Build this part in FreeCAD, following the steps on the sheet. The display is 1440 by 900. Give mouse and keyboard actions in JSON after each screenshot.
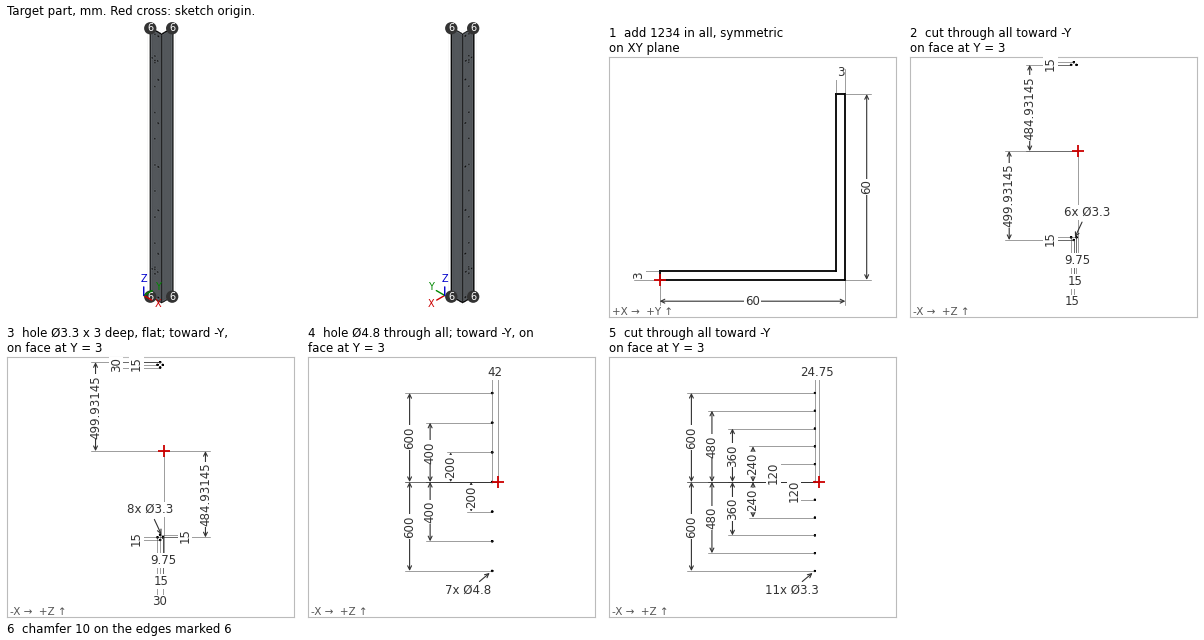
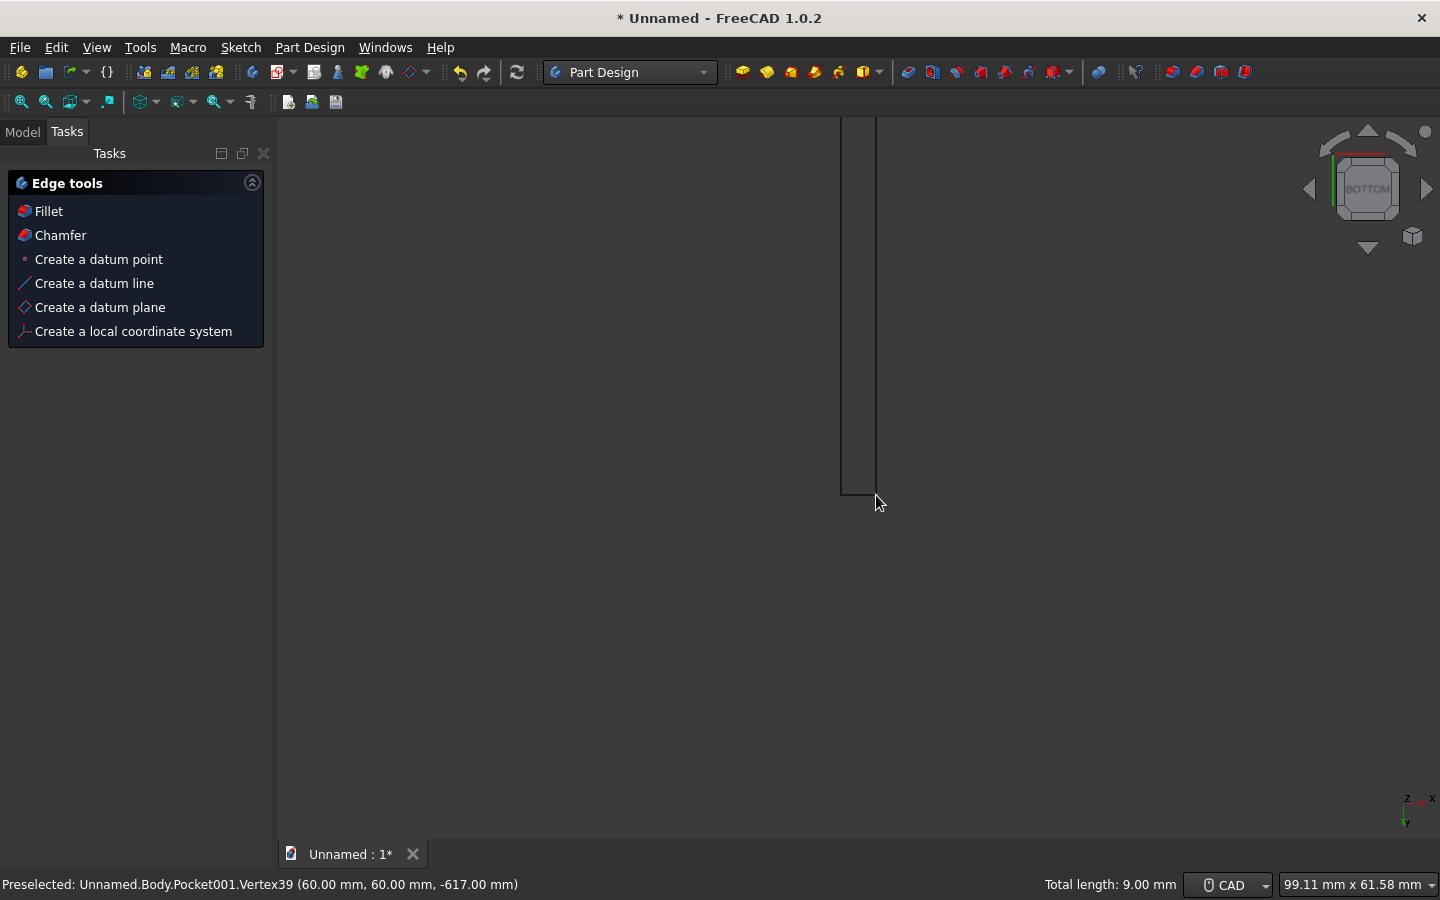
{"action": "left_click", "coordinate": [859, 494], "text": "ctrl"}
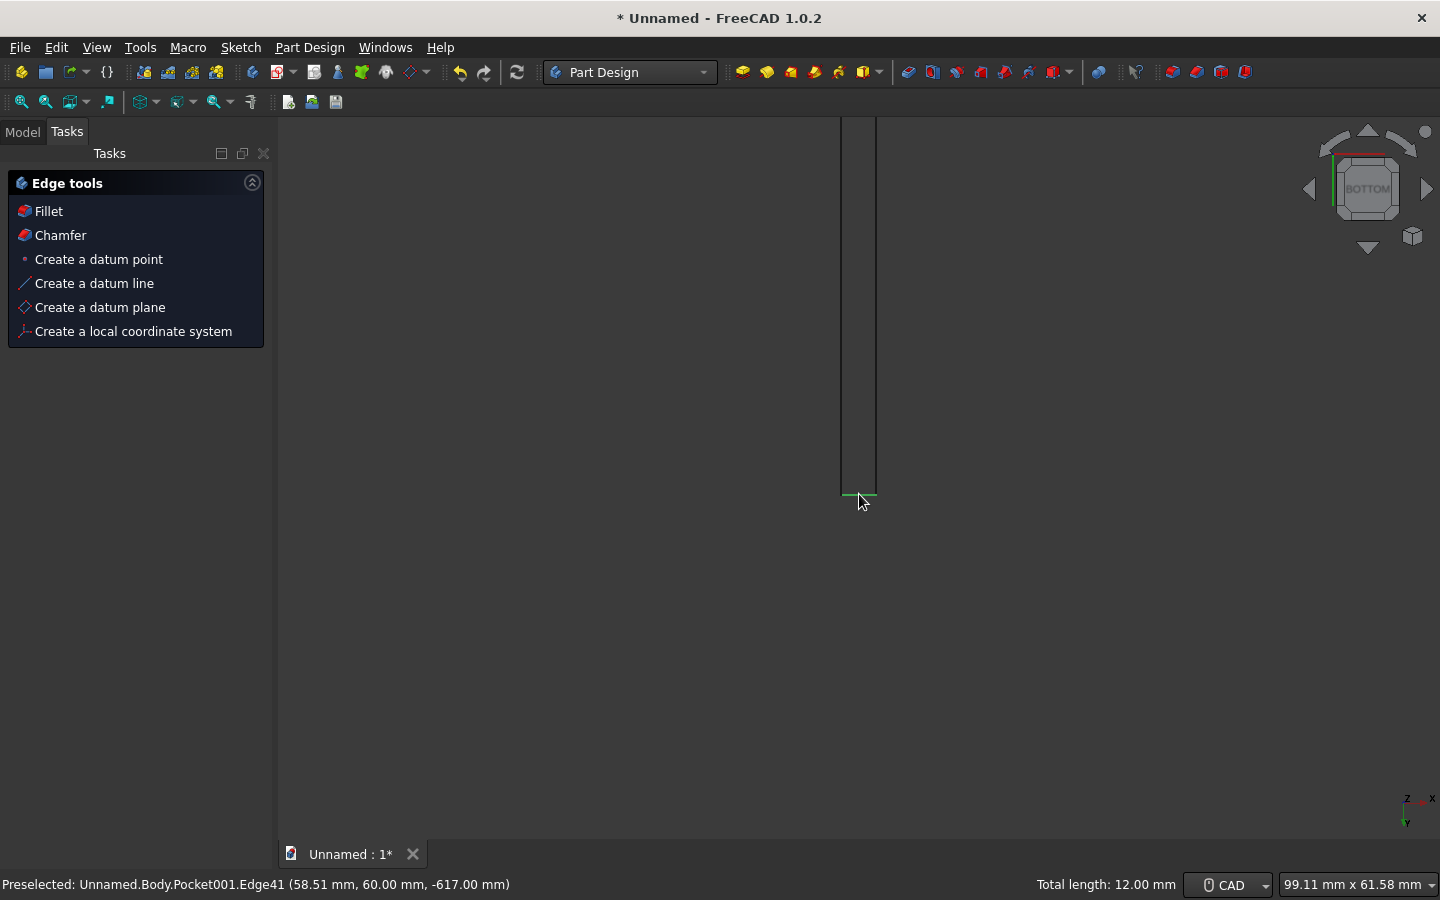
{"action": "key", "text": "v 1"}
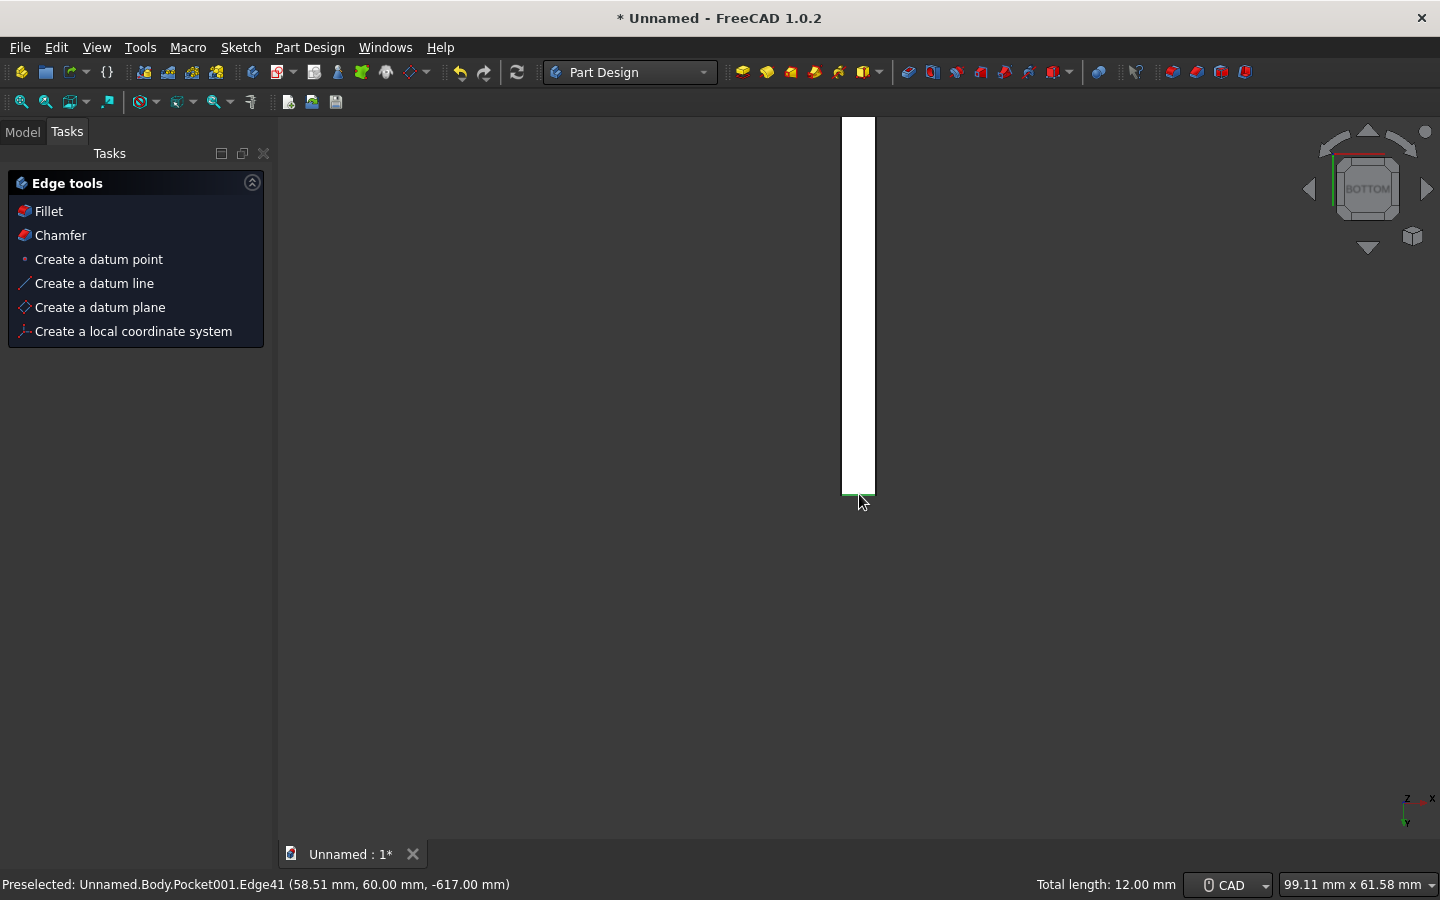
{"action": "left_click", "coordinate": [1198, 72]}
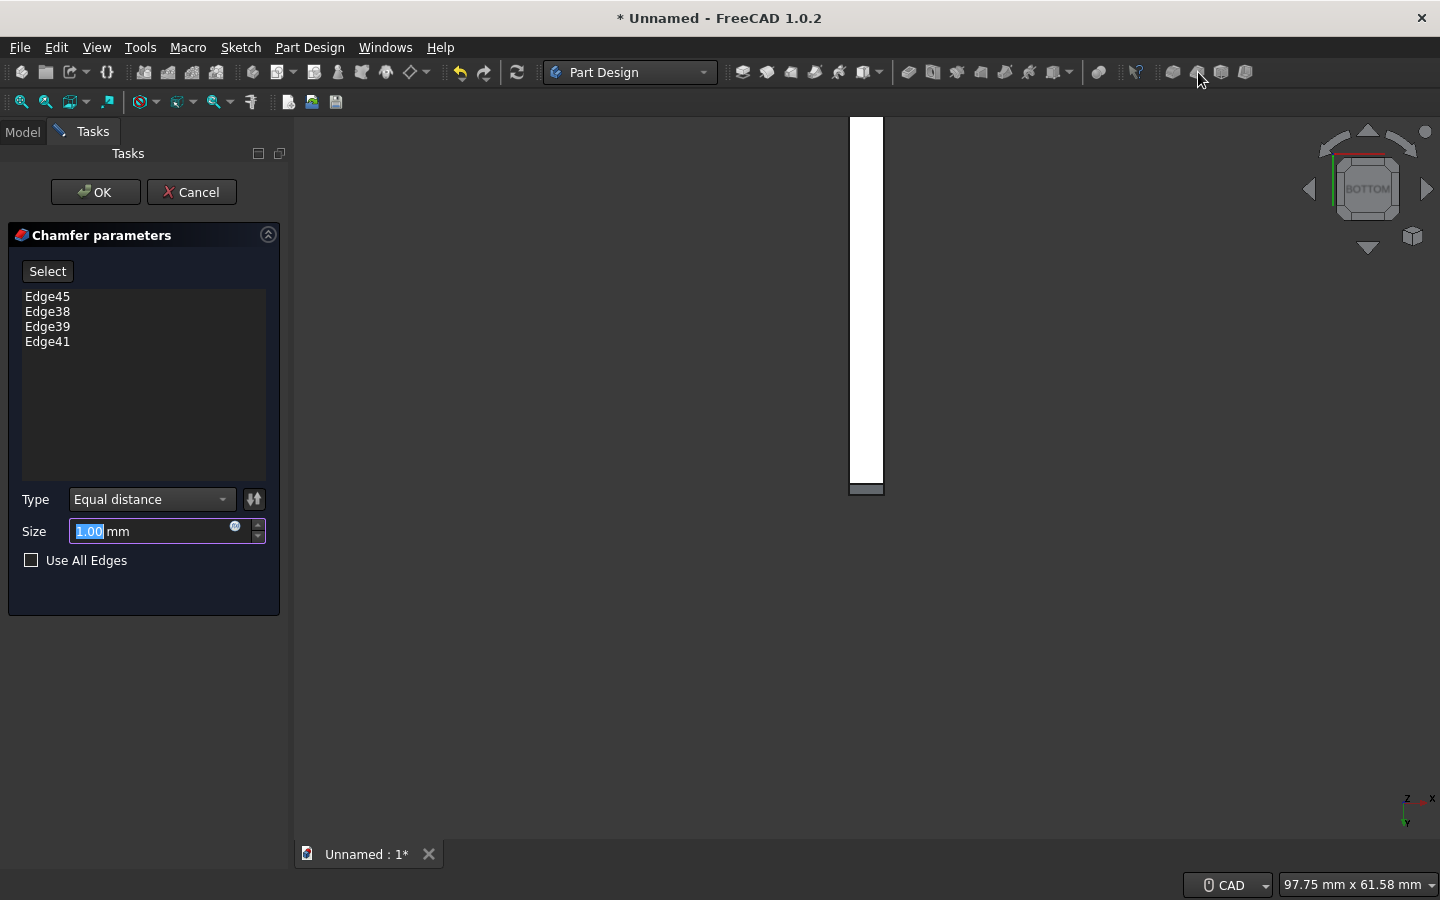
{"action": "type", "text": "10"}
{"action": "key", "text": "Tab"}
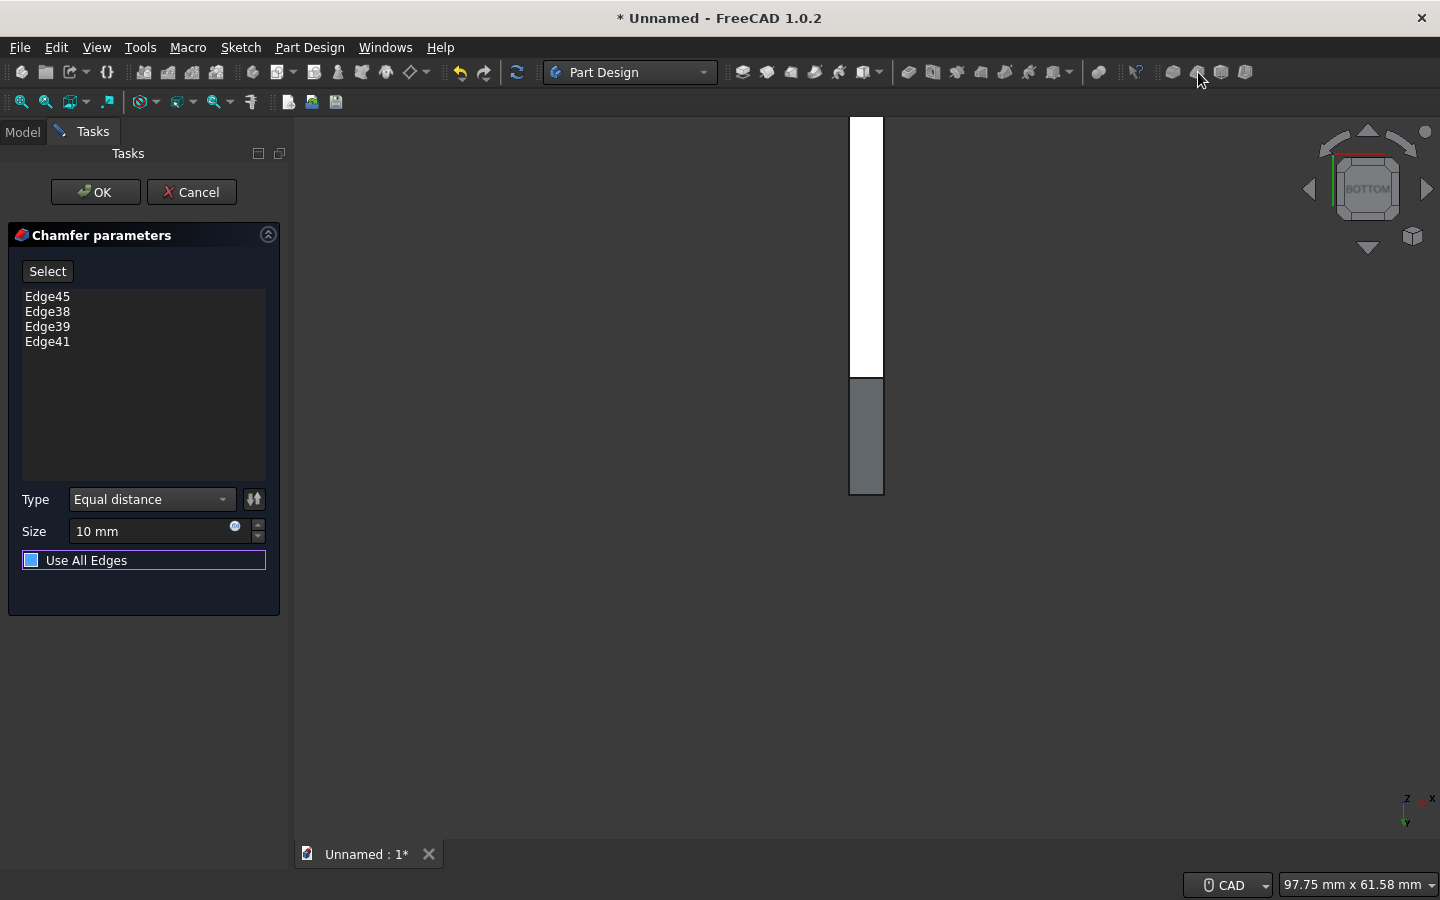
{"action": "left_click", "coordinate": [96, 192]}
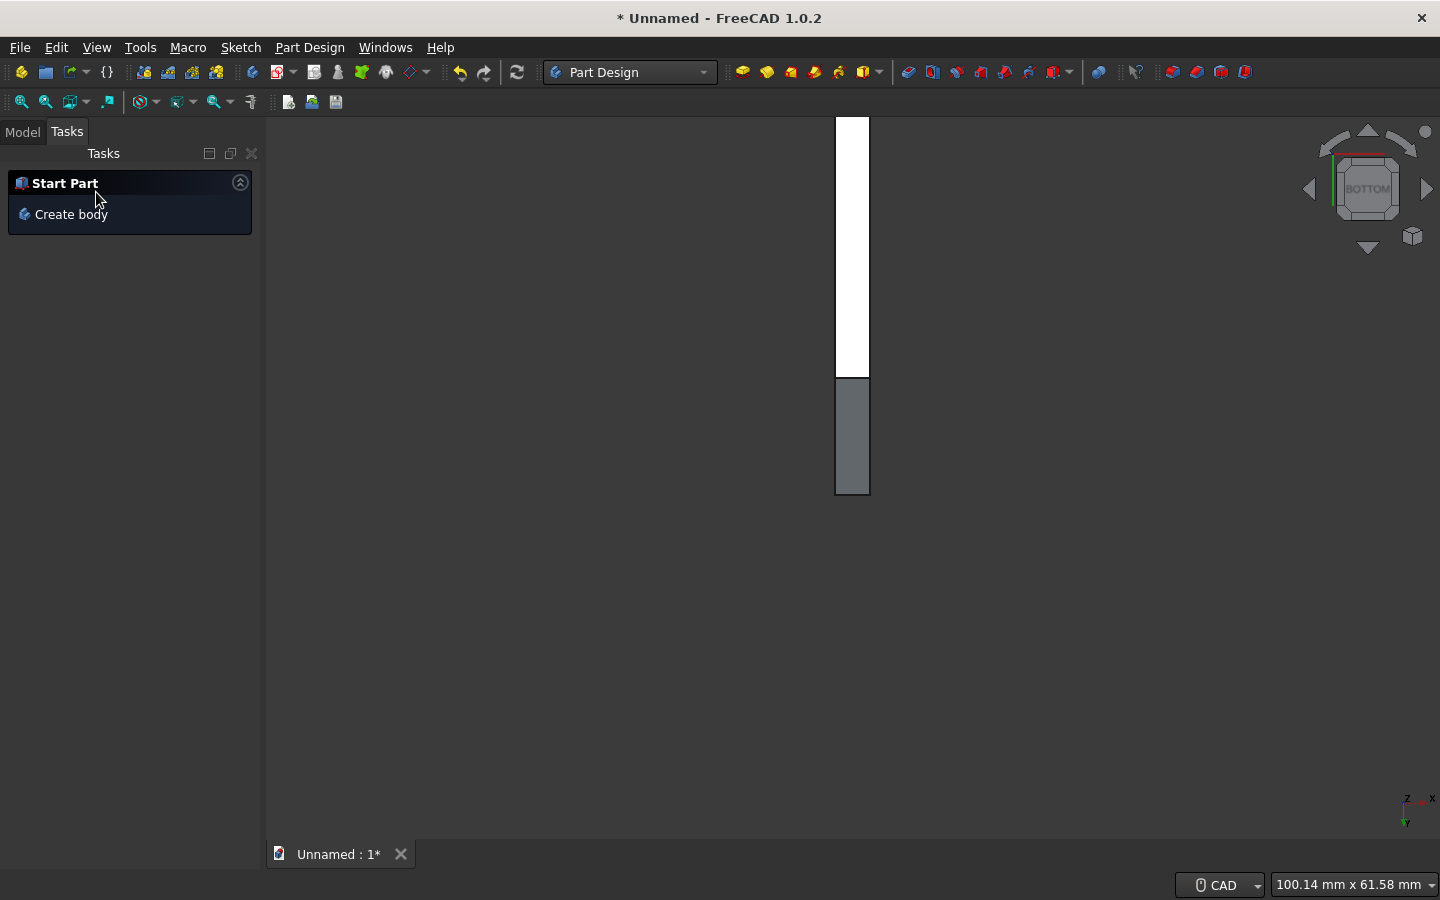
{"action": "key", "text": "0"}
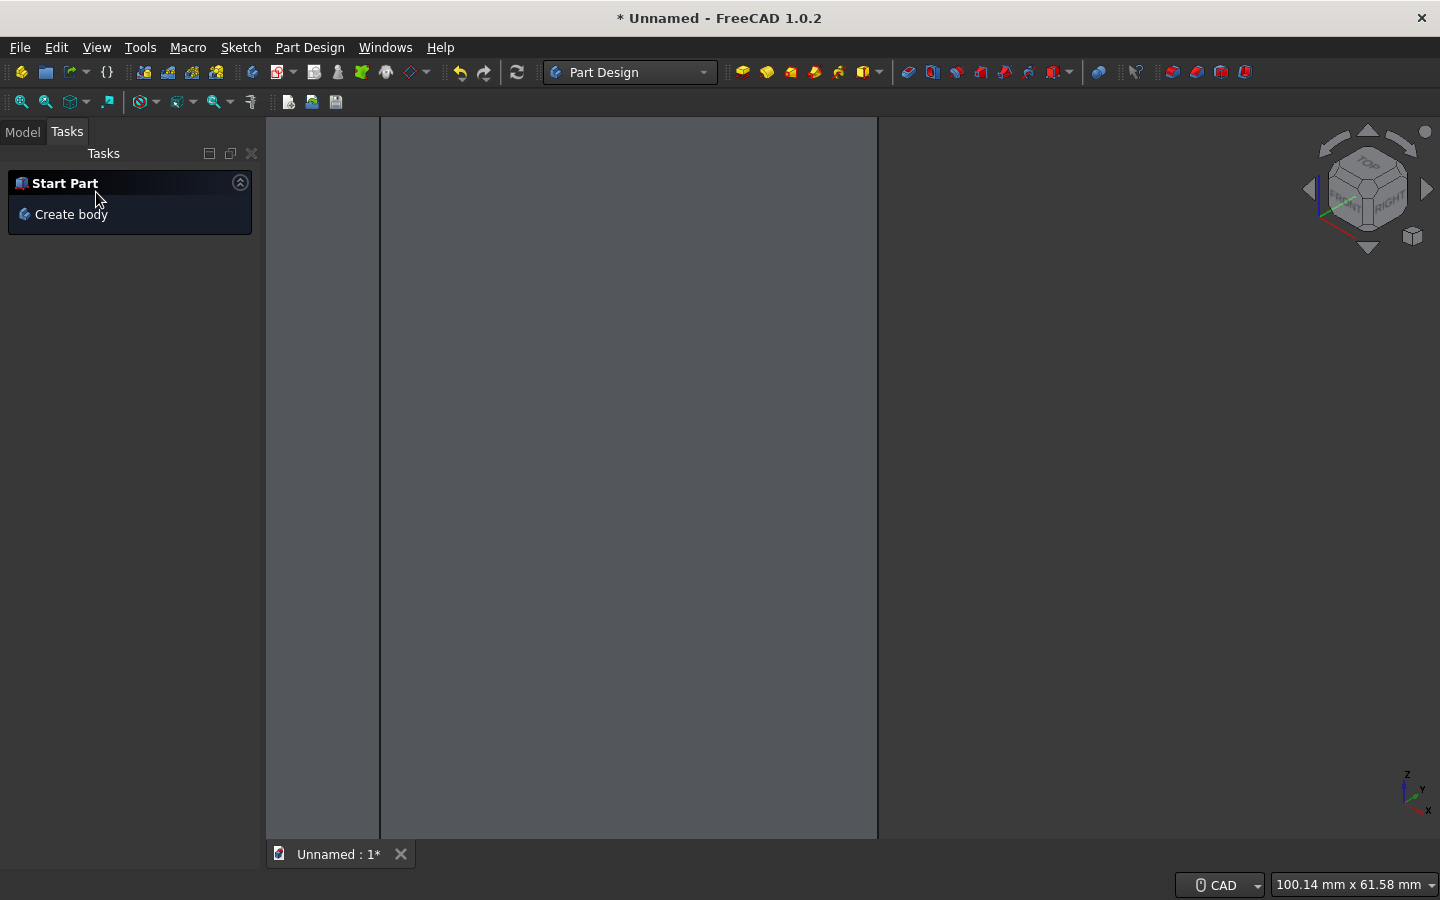
{"action": "left_click", "coordinate": [22, 102]}